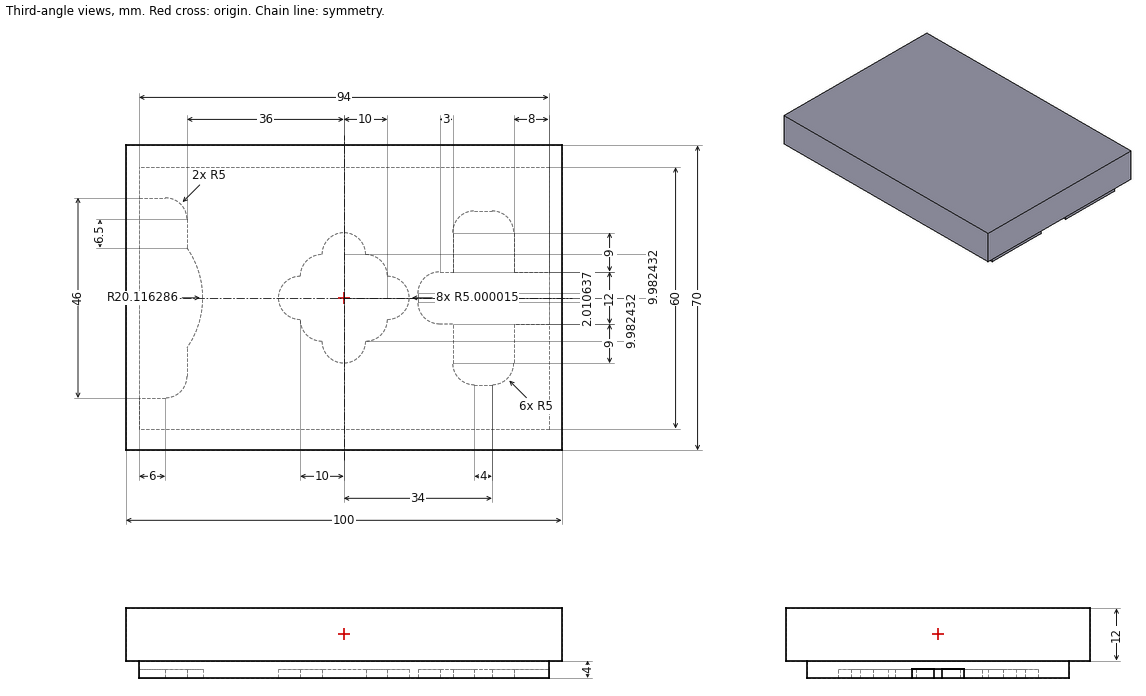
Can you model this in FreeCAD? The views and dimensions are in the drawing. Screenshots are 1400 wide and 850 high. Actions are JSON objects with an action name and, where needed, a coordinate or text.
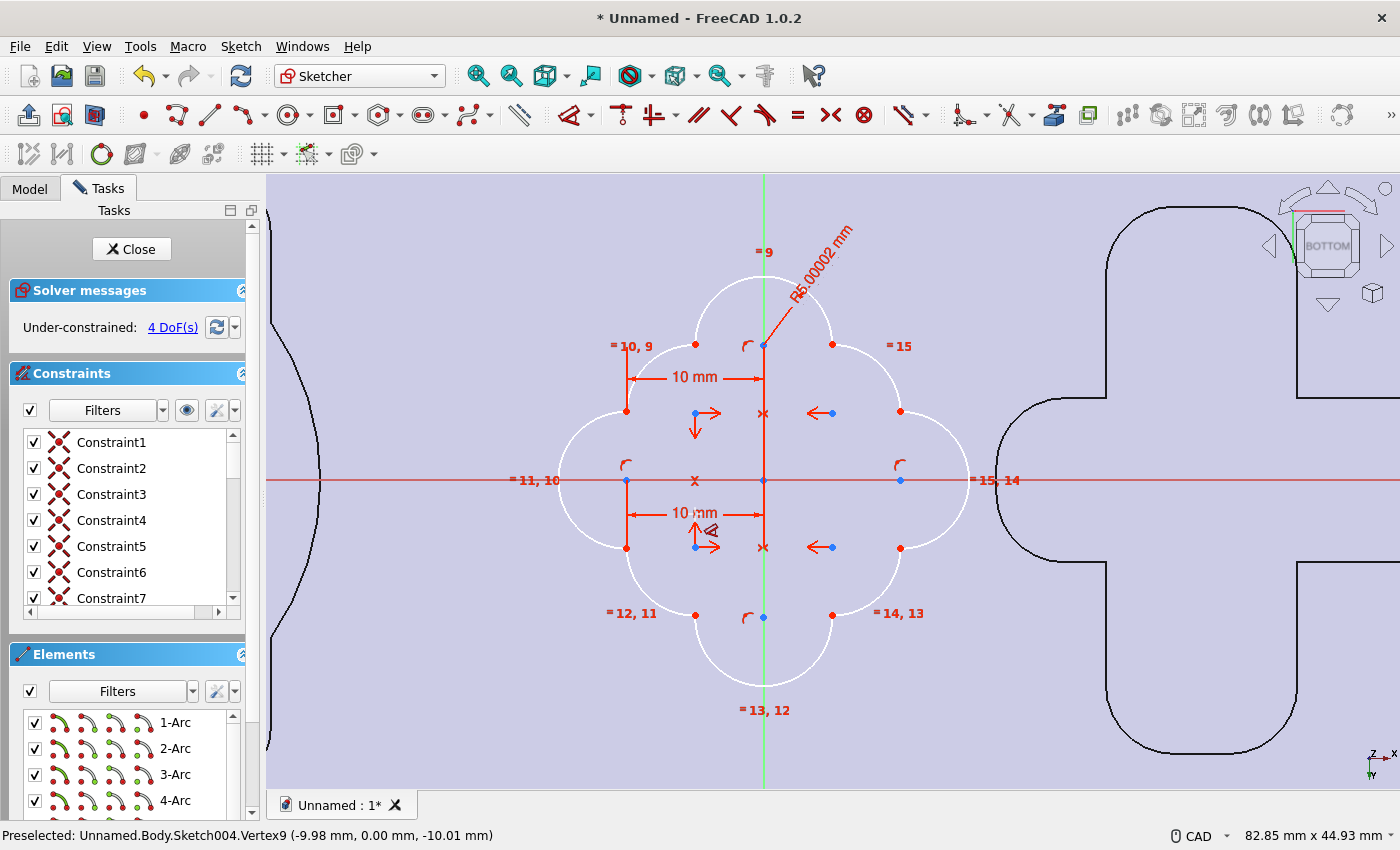
{"action": "left_click", "coordinate": [901, 480]}
{"action": "left_click", "coordinate": [832, 514]}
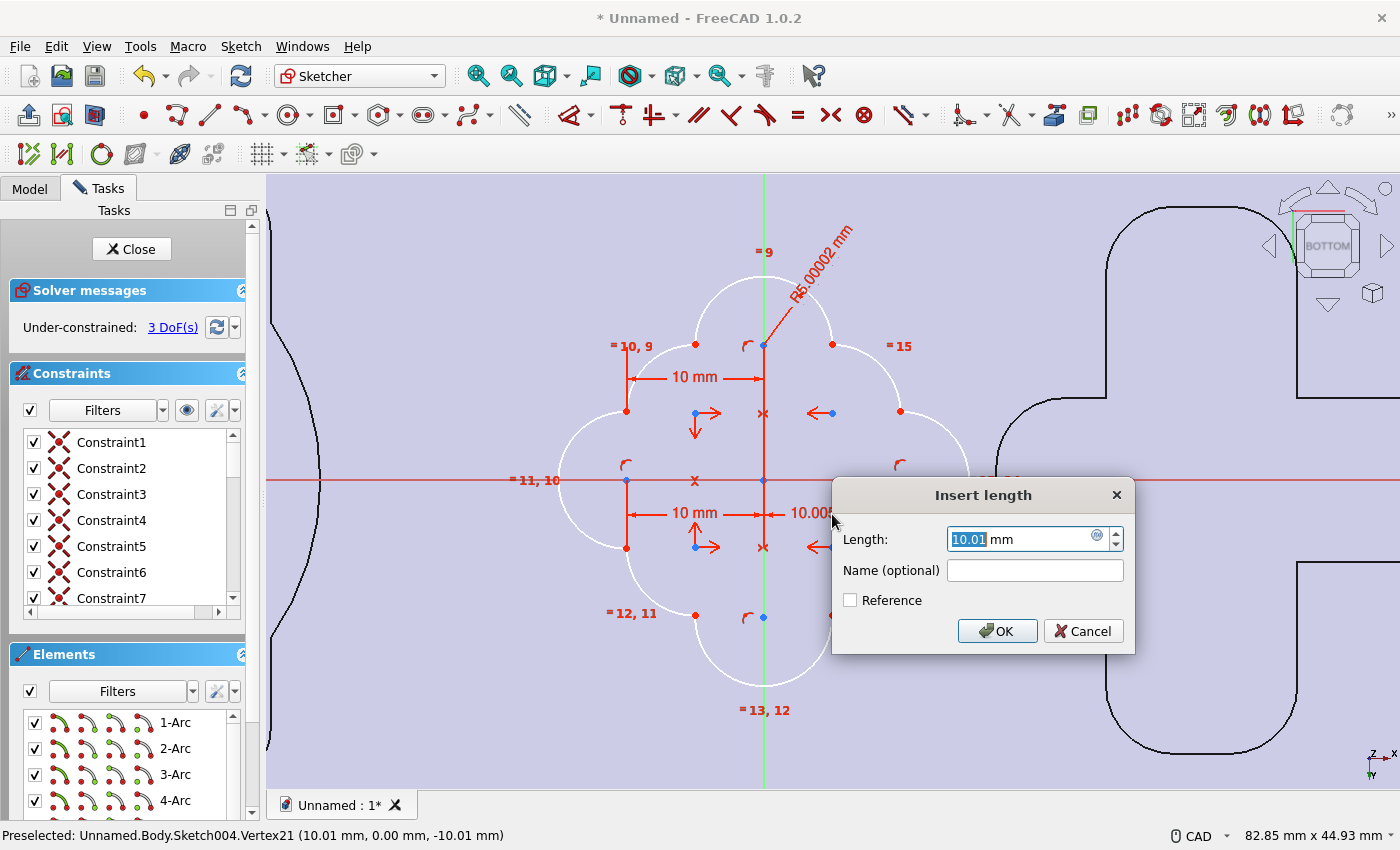
{"action": "type", "text": "10"}
{"action": "key", "text": "Return"}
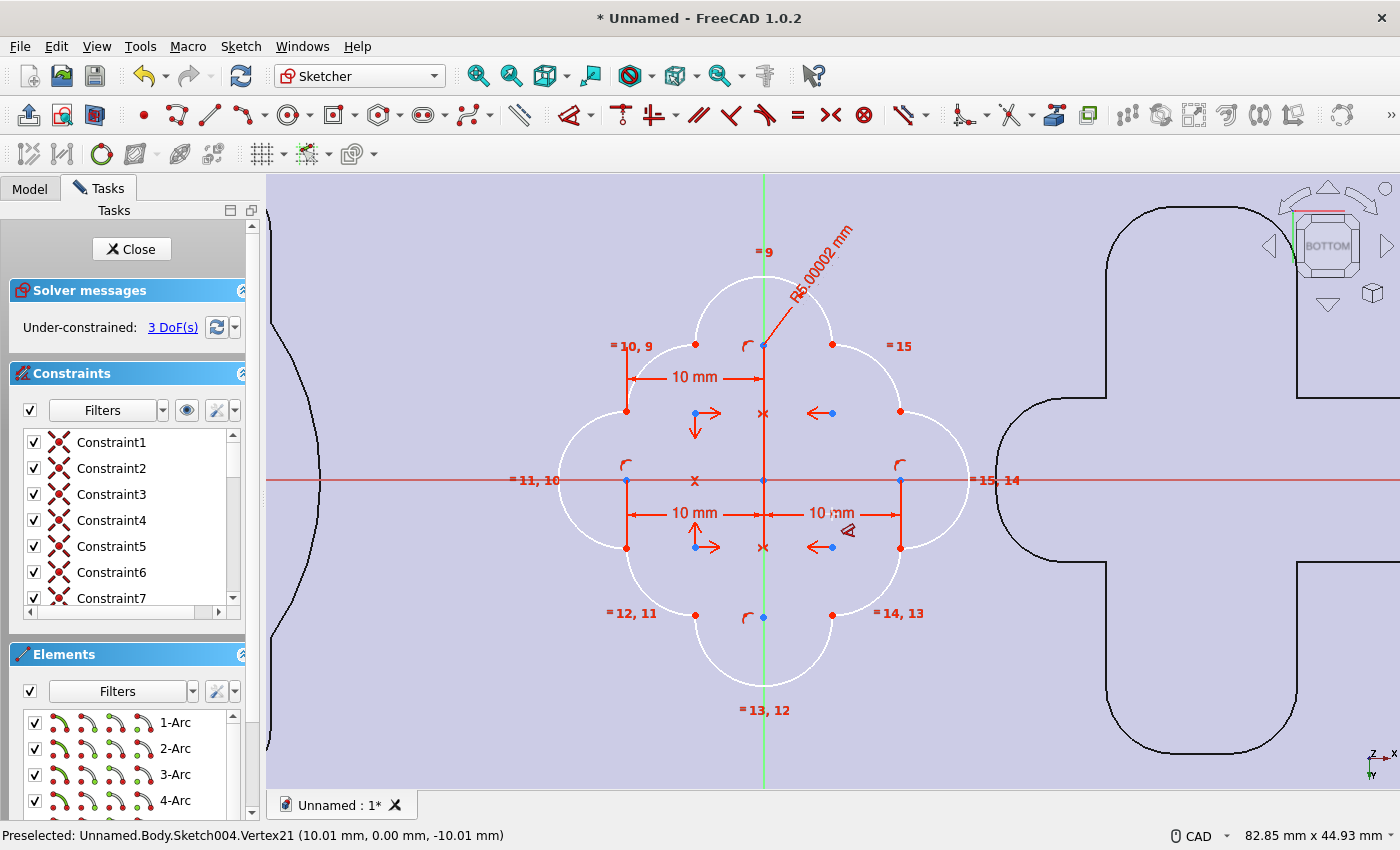
{"action": "left_click", "coordinate": [832, 345]}
{"action": "left_click", "coordinate": [866, 413]}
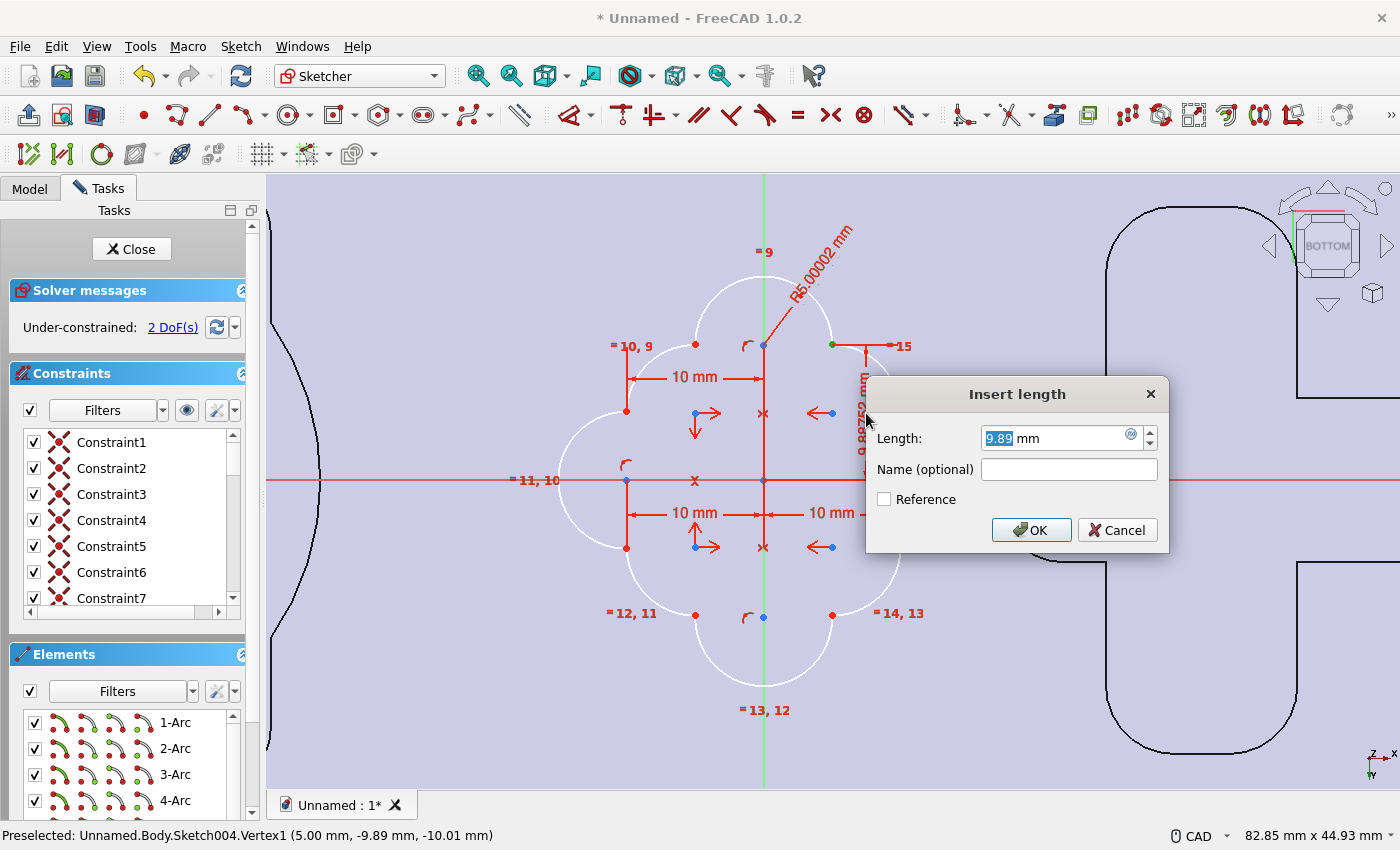
{"action": "type", "text": "9.982432"}
{"action": "key", "text": "Return"}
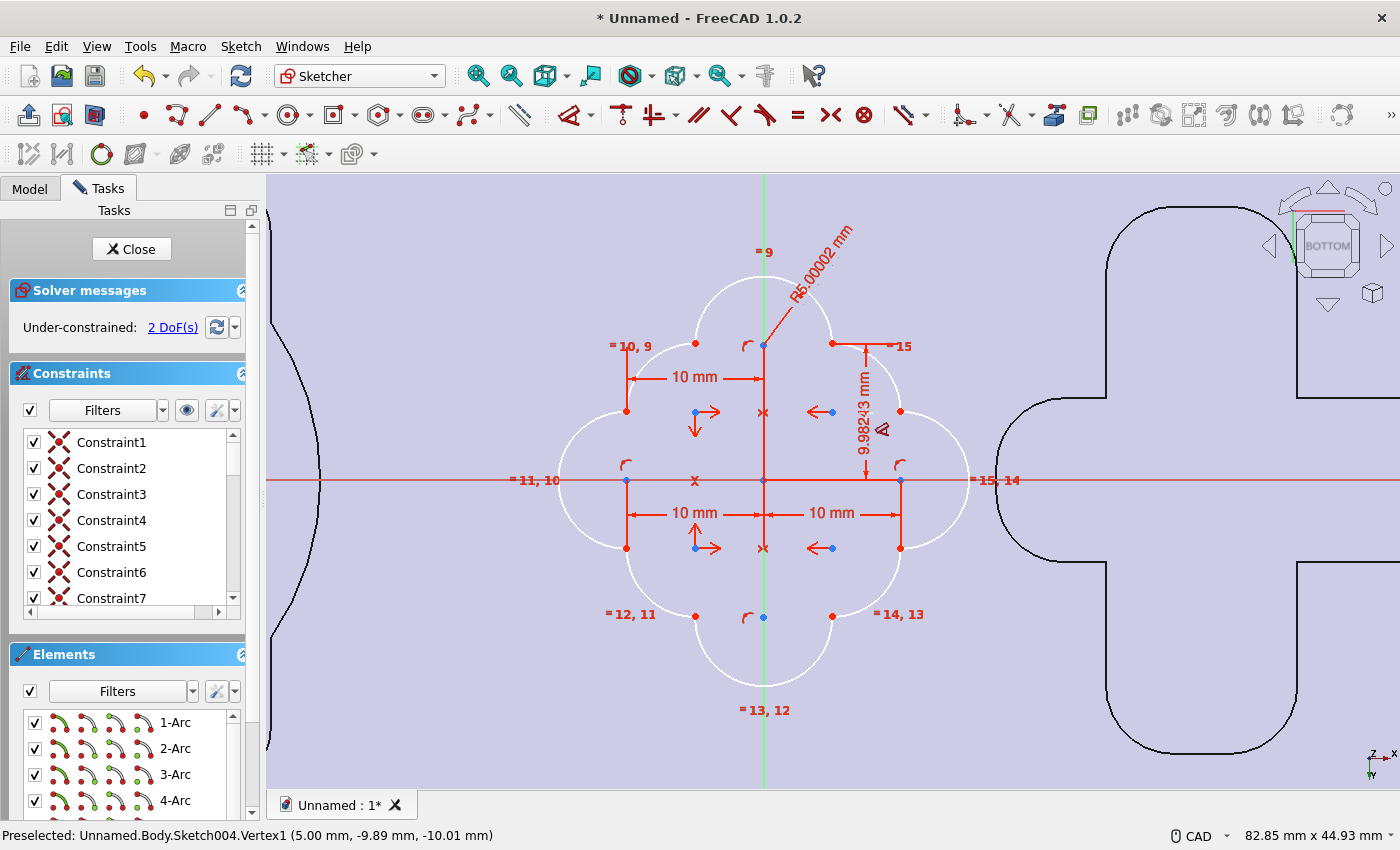
{"action": "left_click", "coordinate": [764, 345]}
{"action": "left_click", "coordinate": [798, 382]}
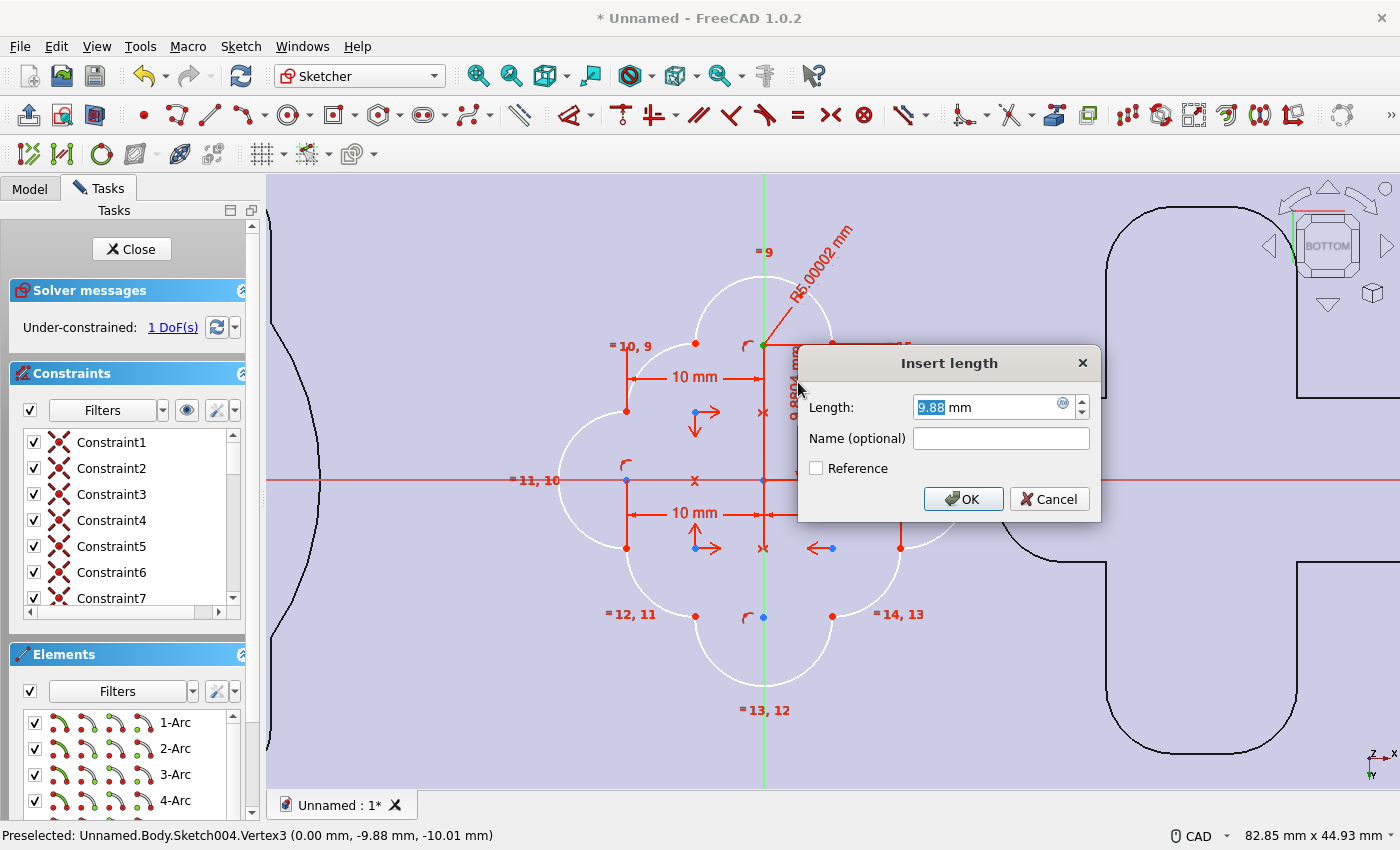
{"action": "type", "text": "9.982432"}
{"action": "key", "text": "Return"}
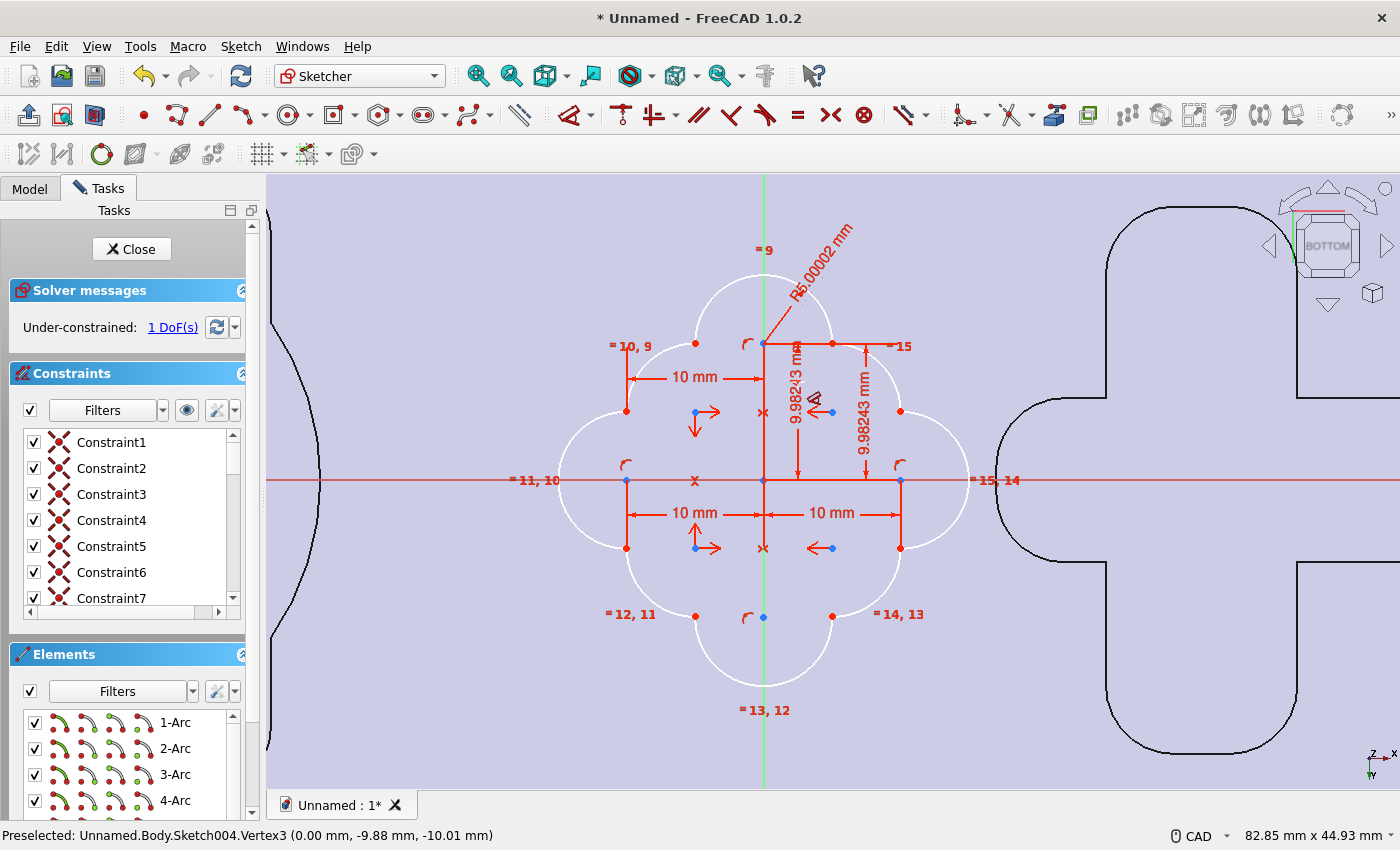
{"action": "left_click", "coordinate": [764, 618]}
{"action": "left_click", "coordinate": [798, 549]}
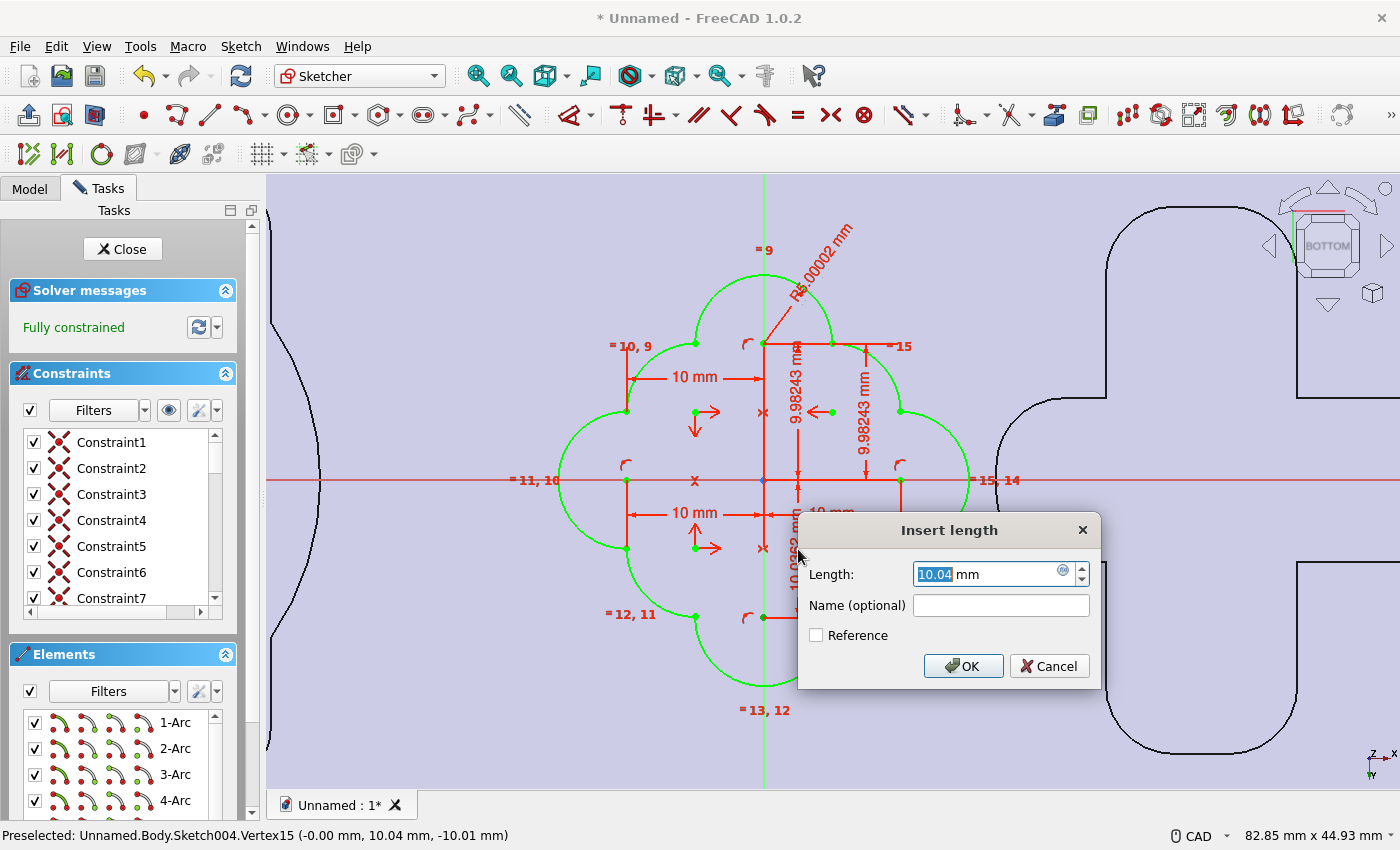
{"action": "type", "text": "9.982432"}
{"action": "key", "text": "Return"}
{"action": "key", "text": "Escape"}